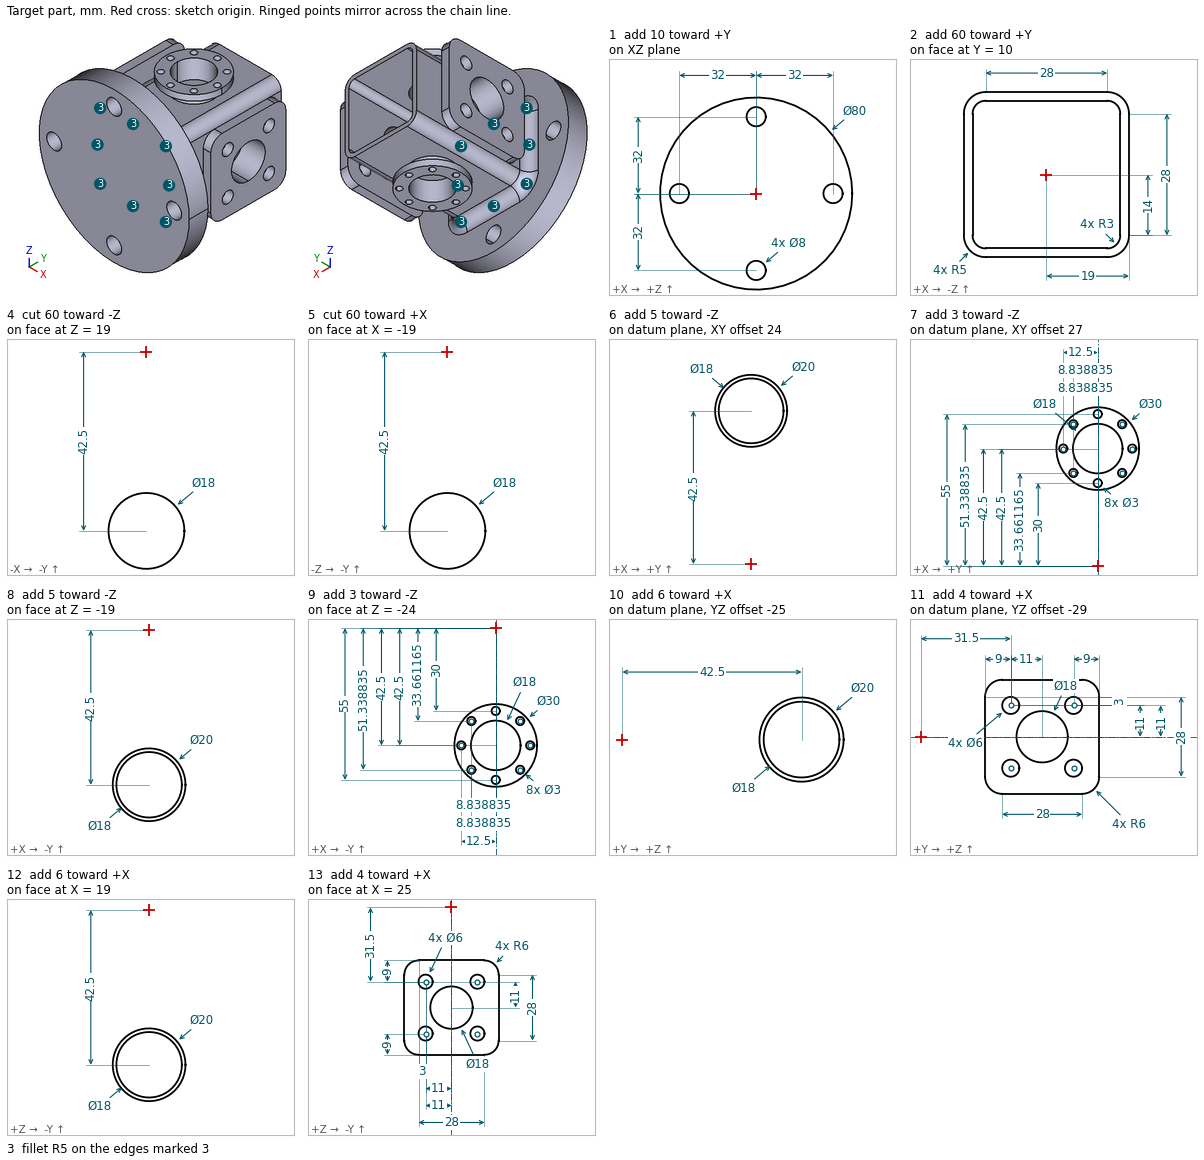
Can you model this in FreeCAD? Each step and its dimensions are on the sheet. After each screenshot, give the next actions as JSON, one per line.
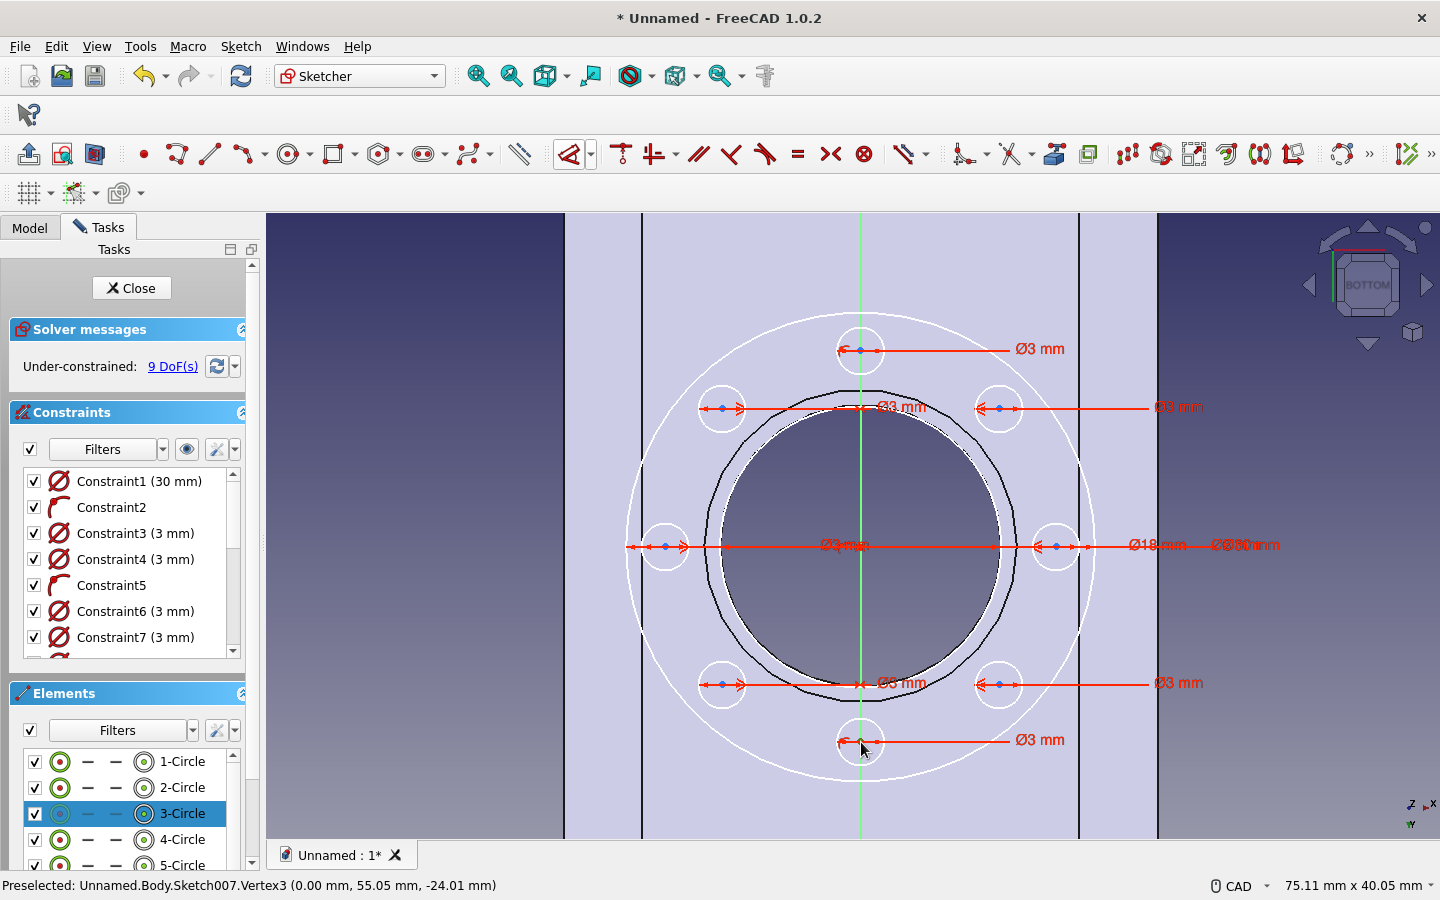
{"action": "key", "text": "i"}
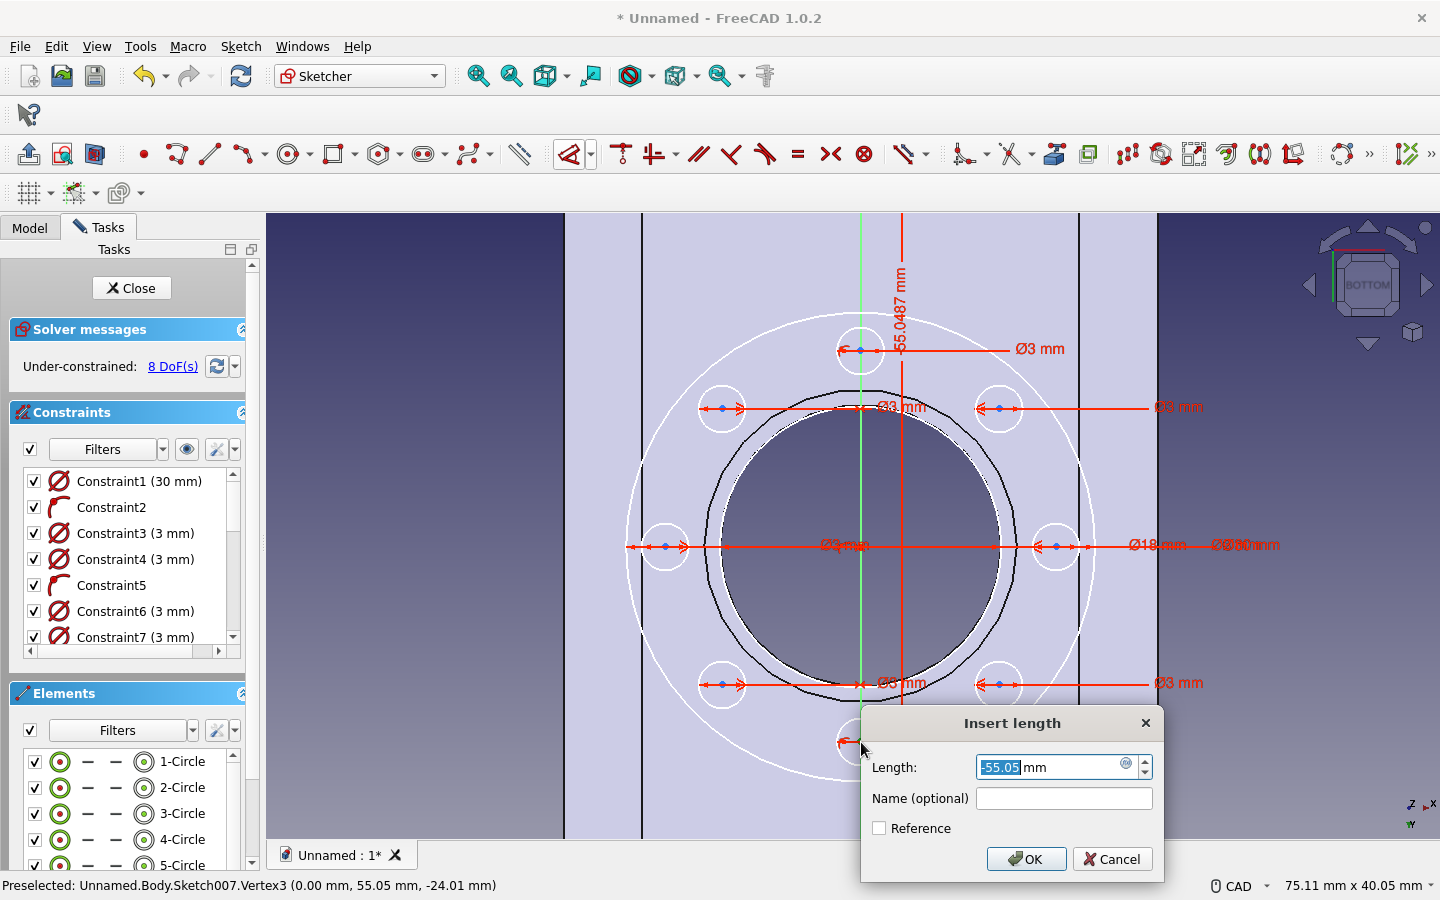
{"action": "type", "text": "-55"}
{"action": "key", "text": "Return"}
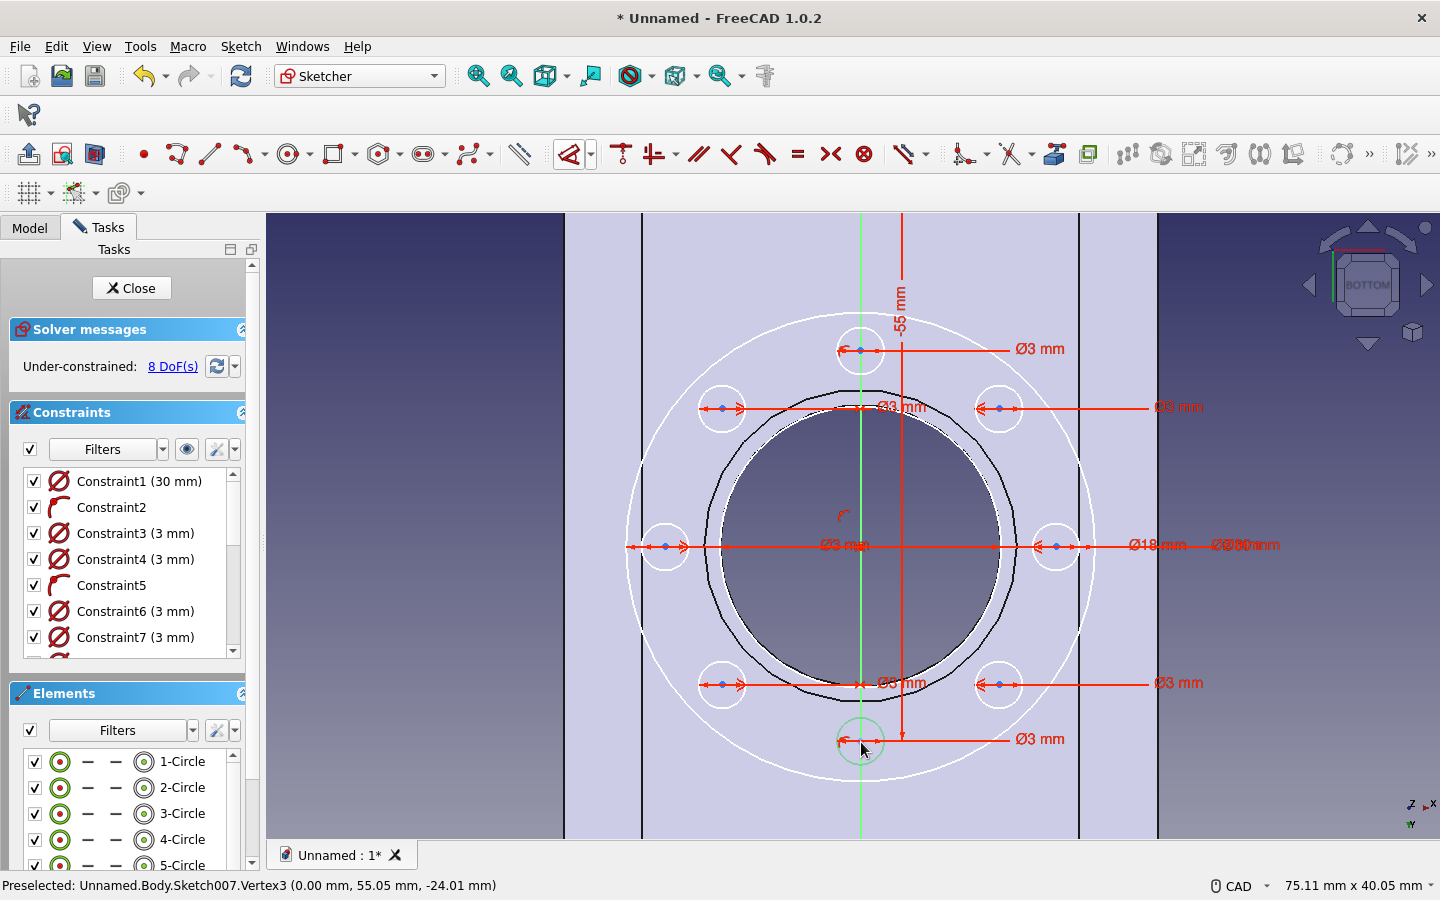
{"action": "left_click", "coordinate": [861, 351]}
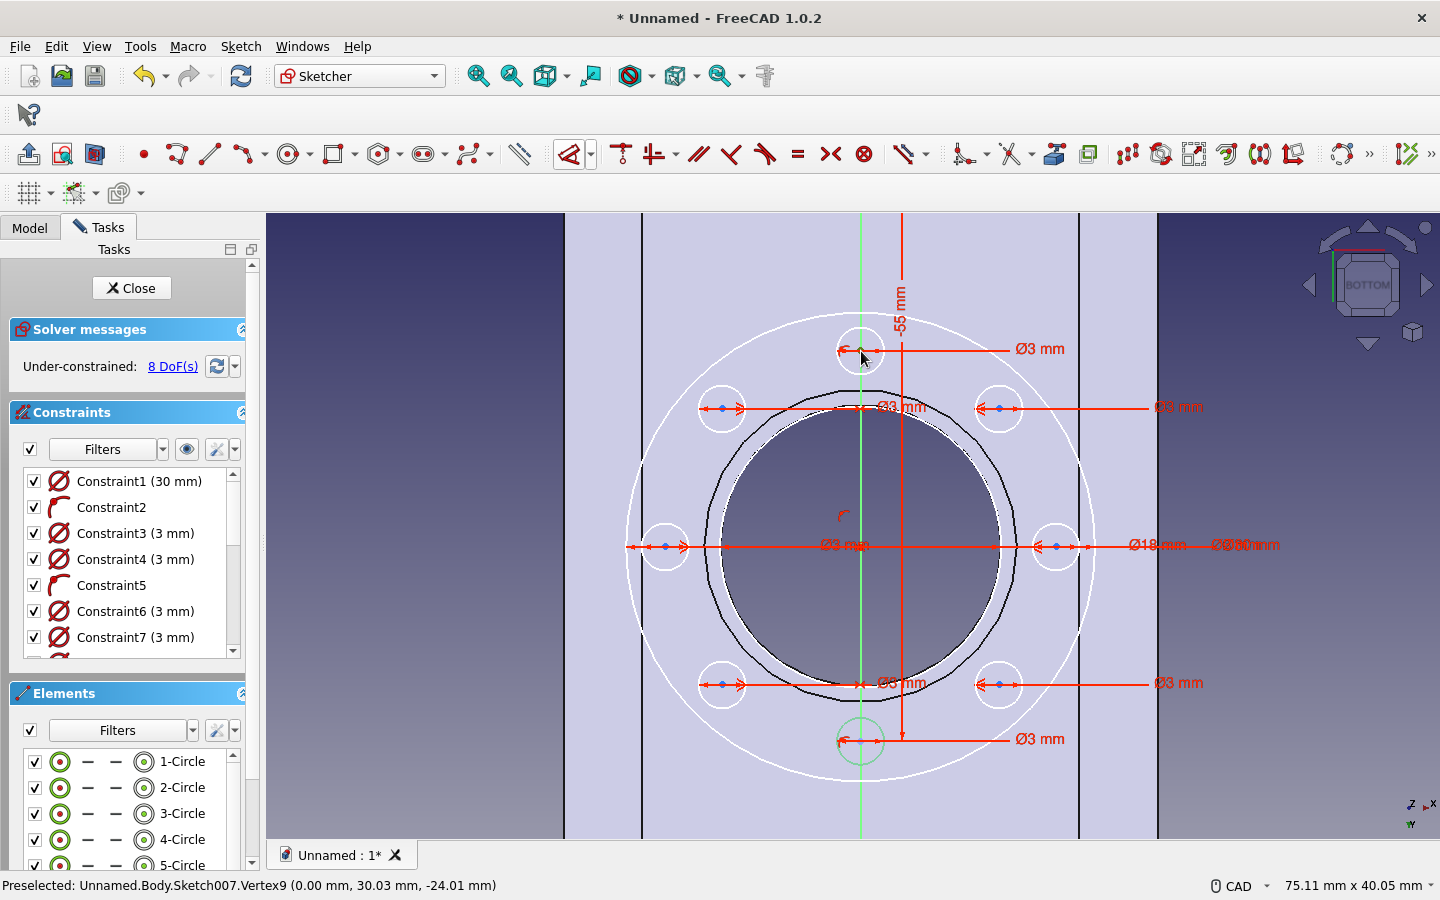
{"action": "key", "text": "i"}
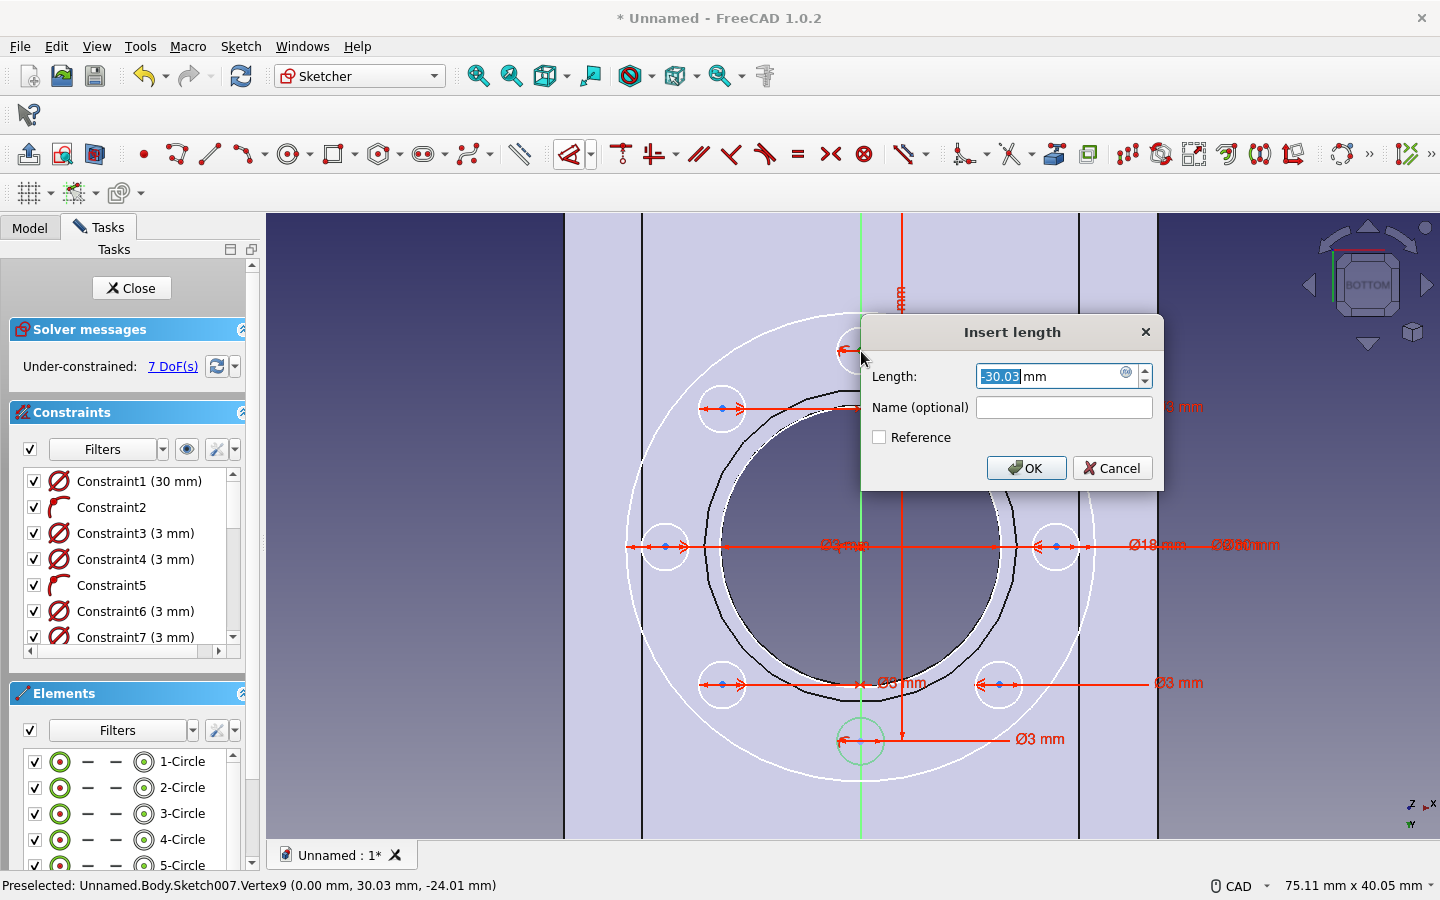
{"action": "type", "text": "-30"}
{"action": "key", "text": "Return"}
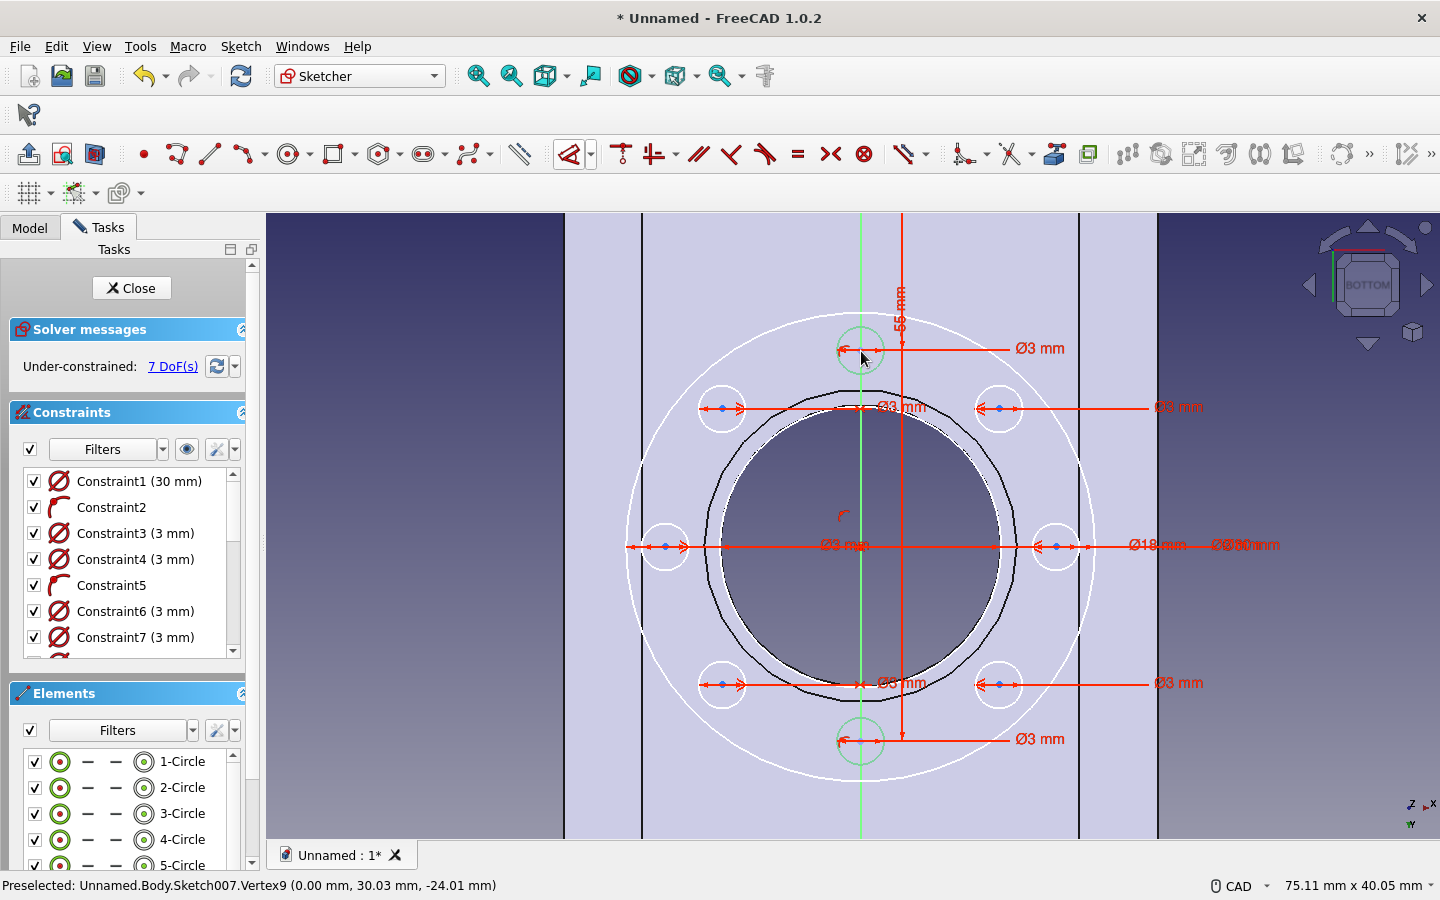
{"action": "left_click", "coordinate": [861, 547]}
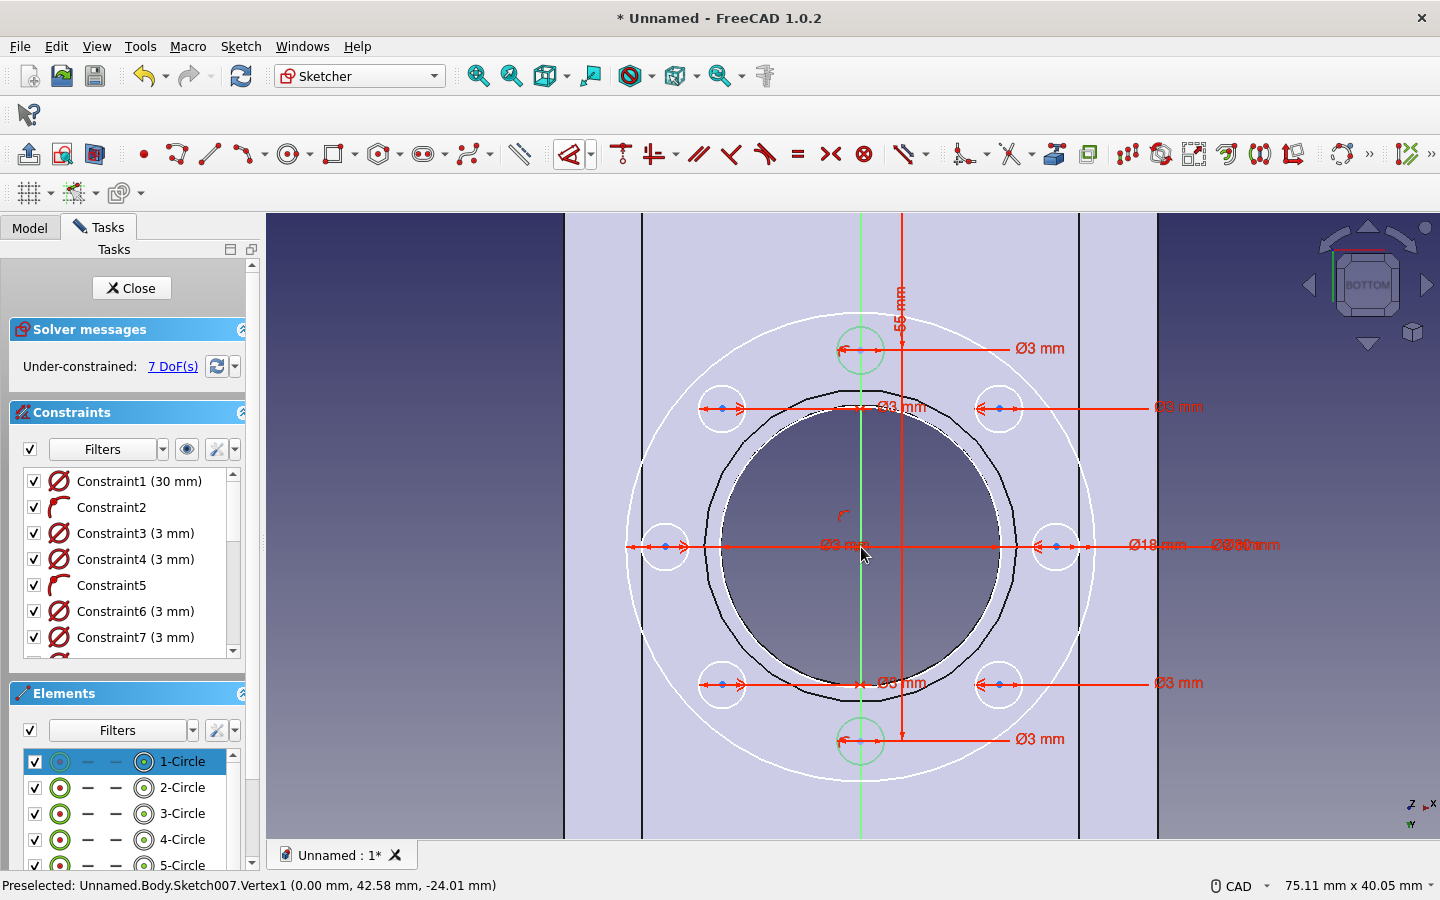
{"action": "key", "text": "i"}